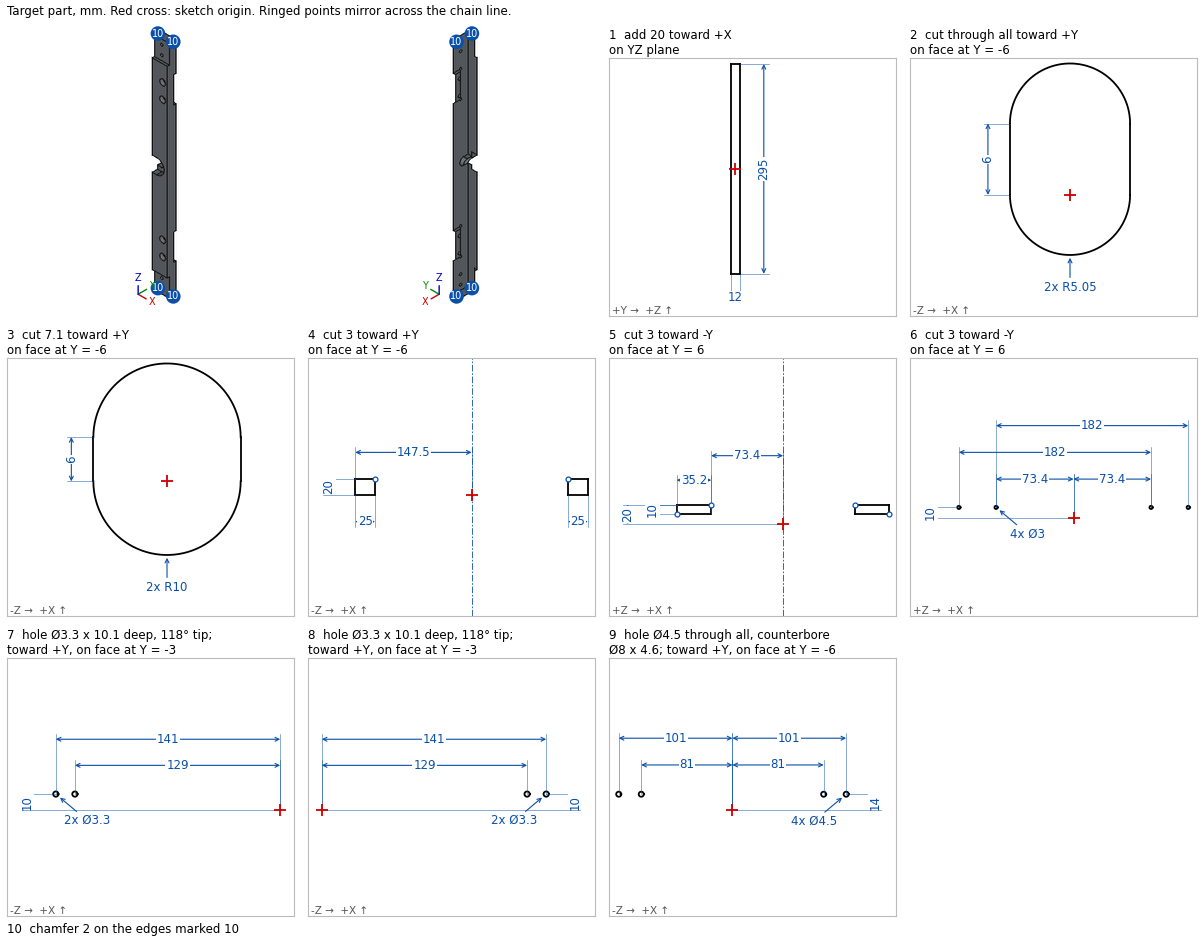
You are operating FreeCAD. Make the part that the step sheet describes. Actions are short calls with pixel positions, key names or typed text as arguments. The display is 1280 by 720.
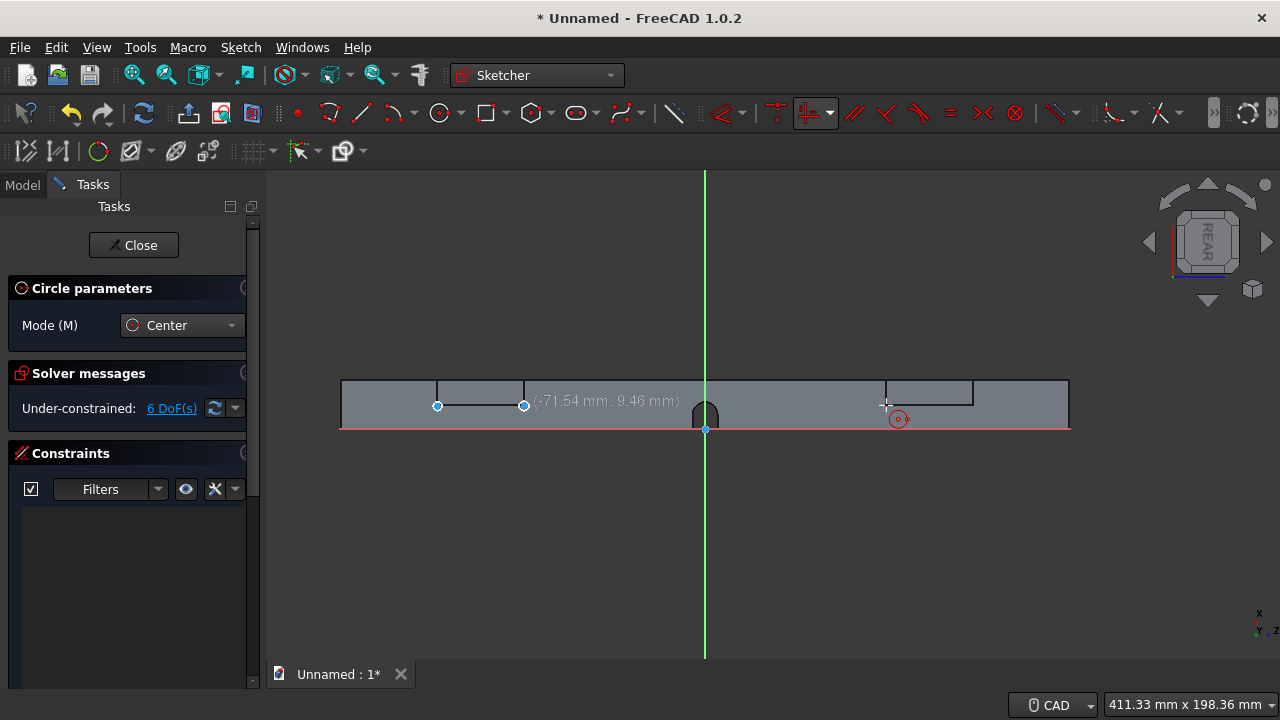
click(886, 405)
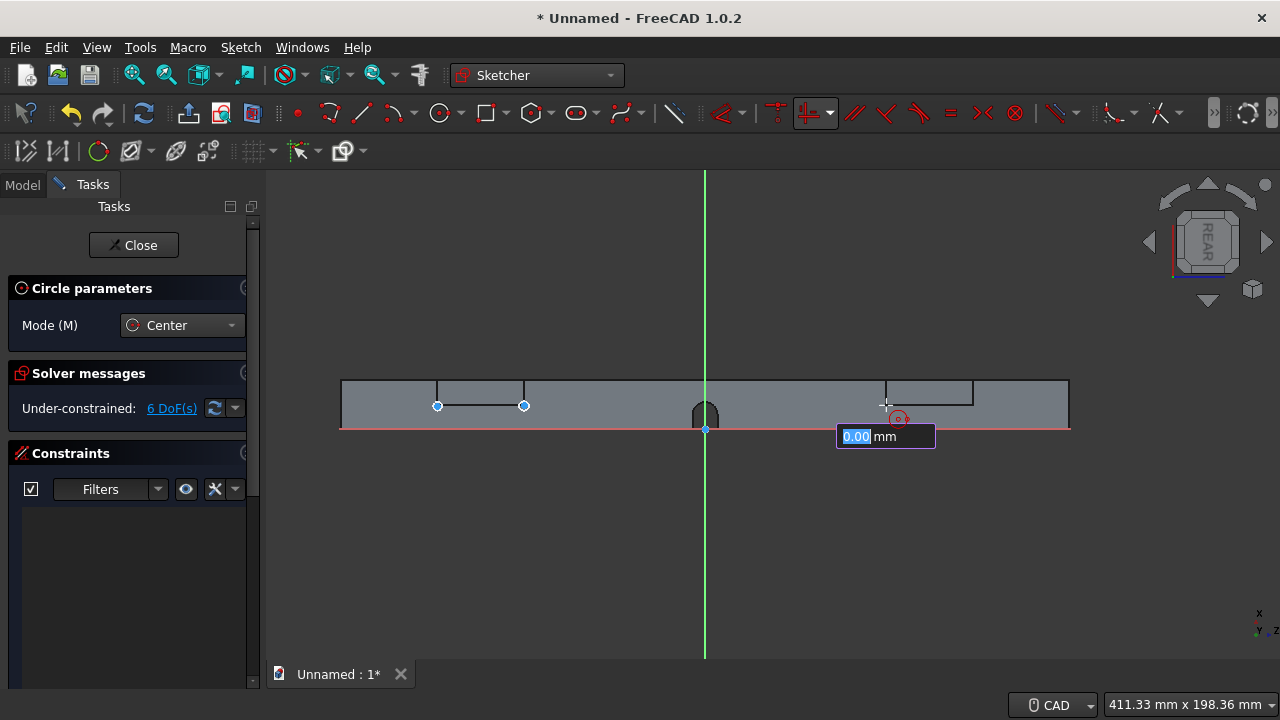
scroll(889, 402, up, 8)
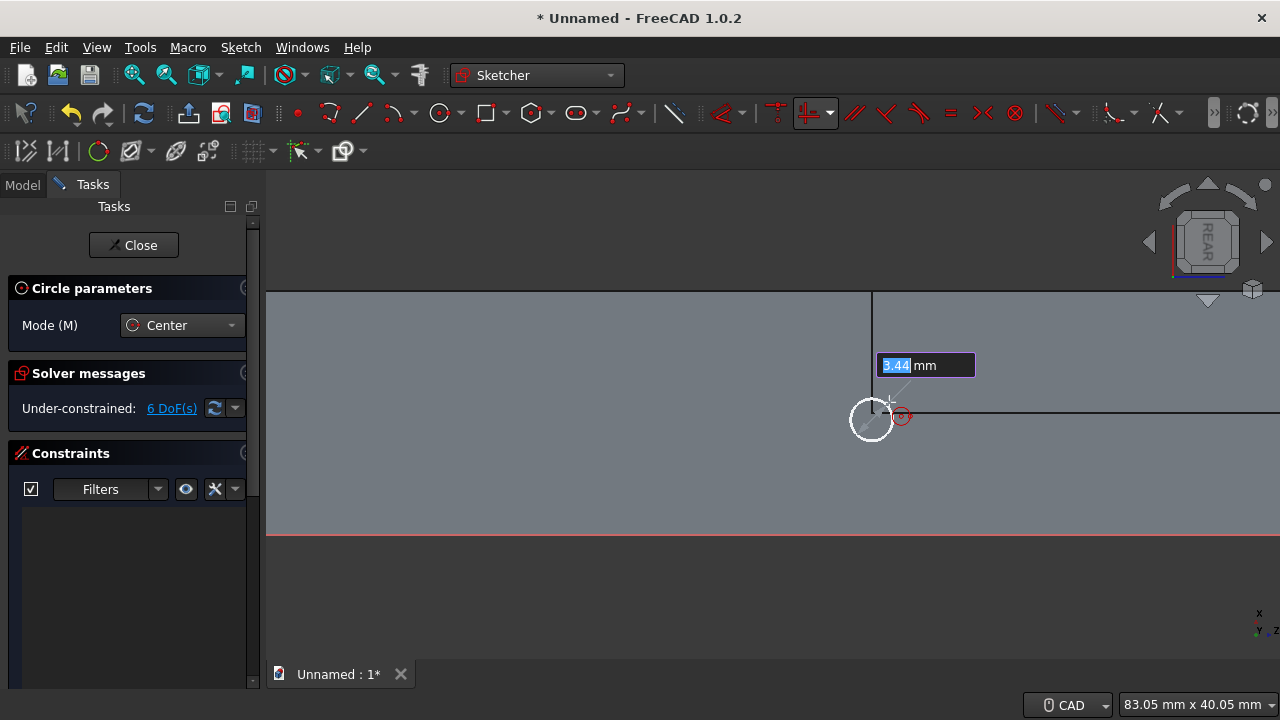
click(885, 400)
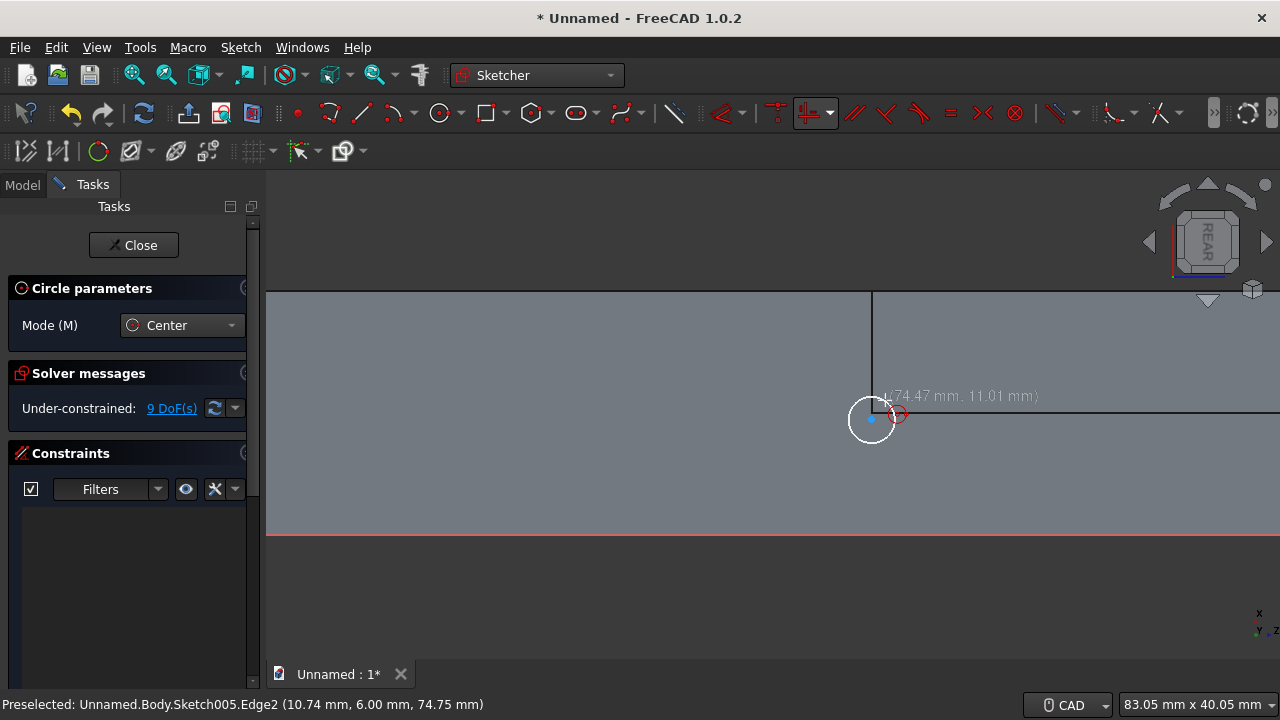
scroll(889, 402, down, 8)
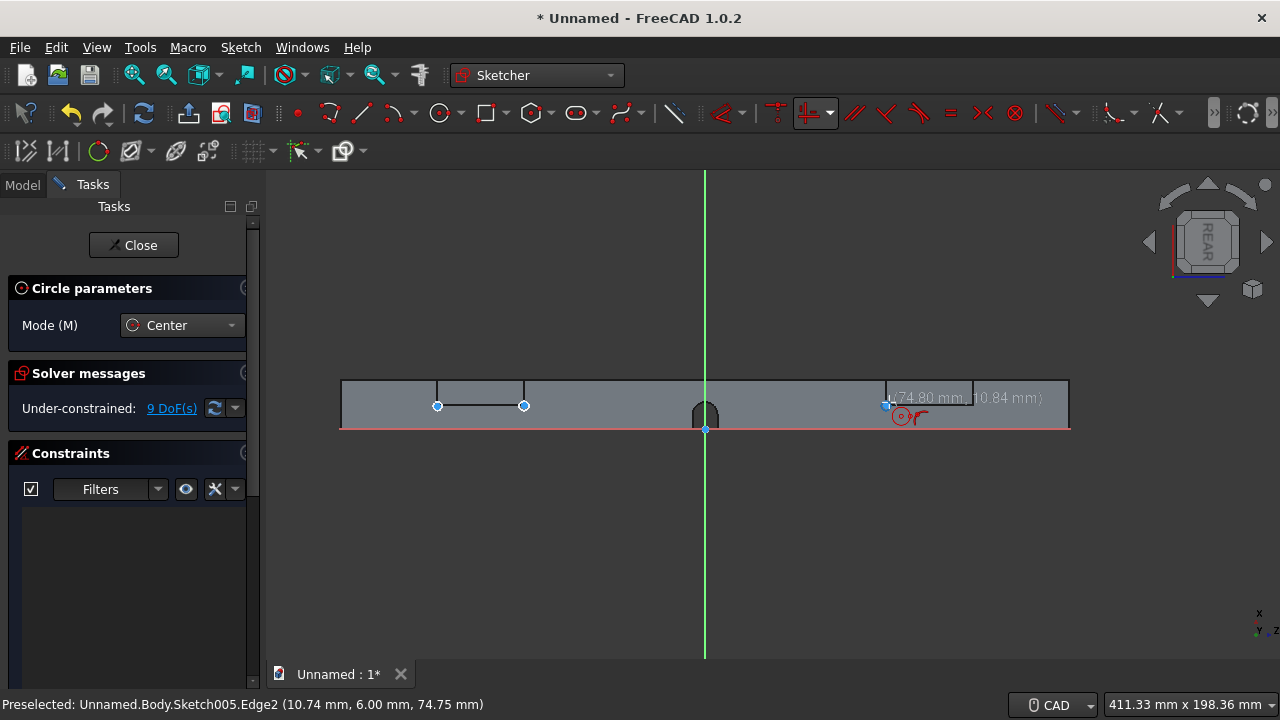
scroll(973, 405, up, 10)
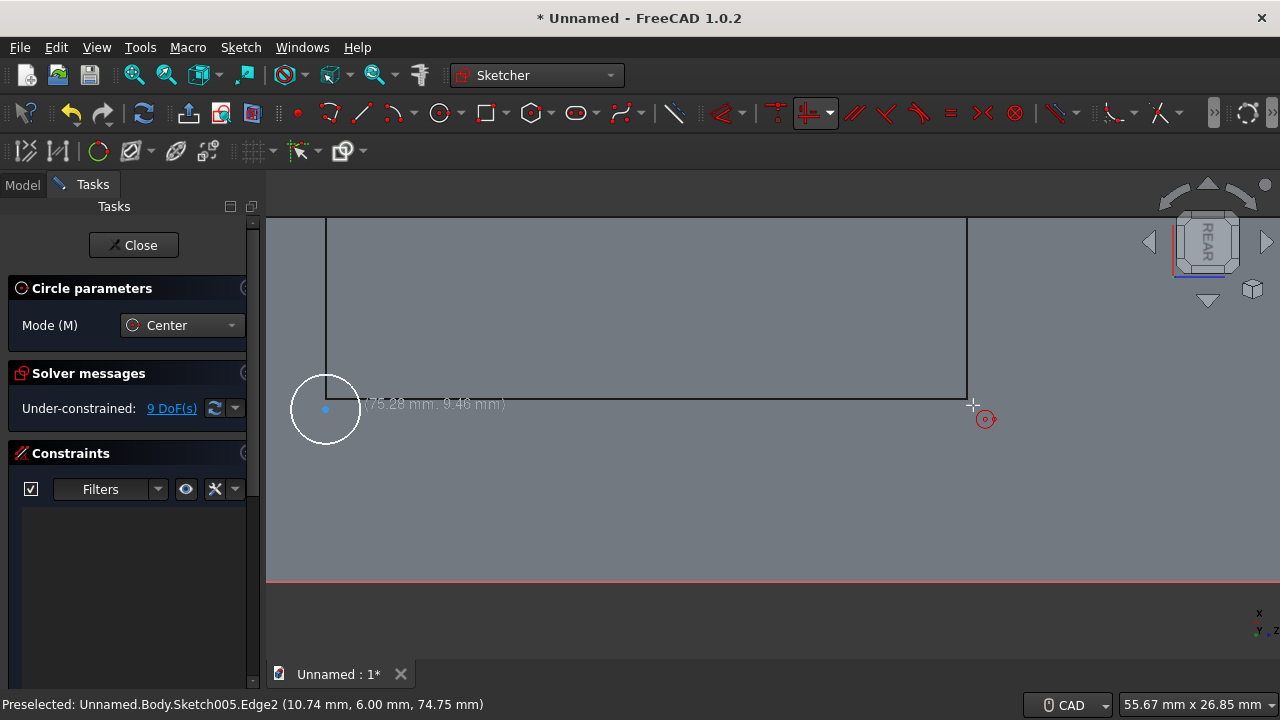
scroll(973, 405, down, 10)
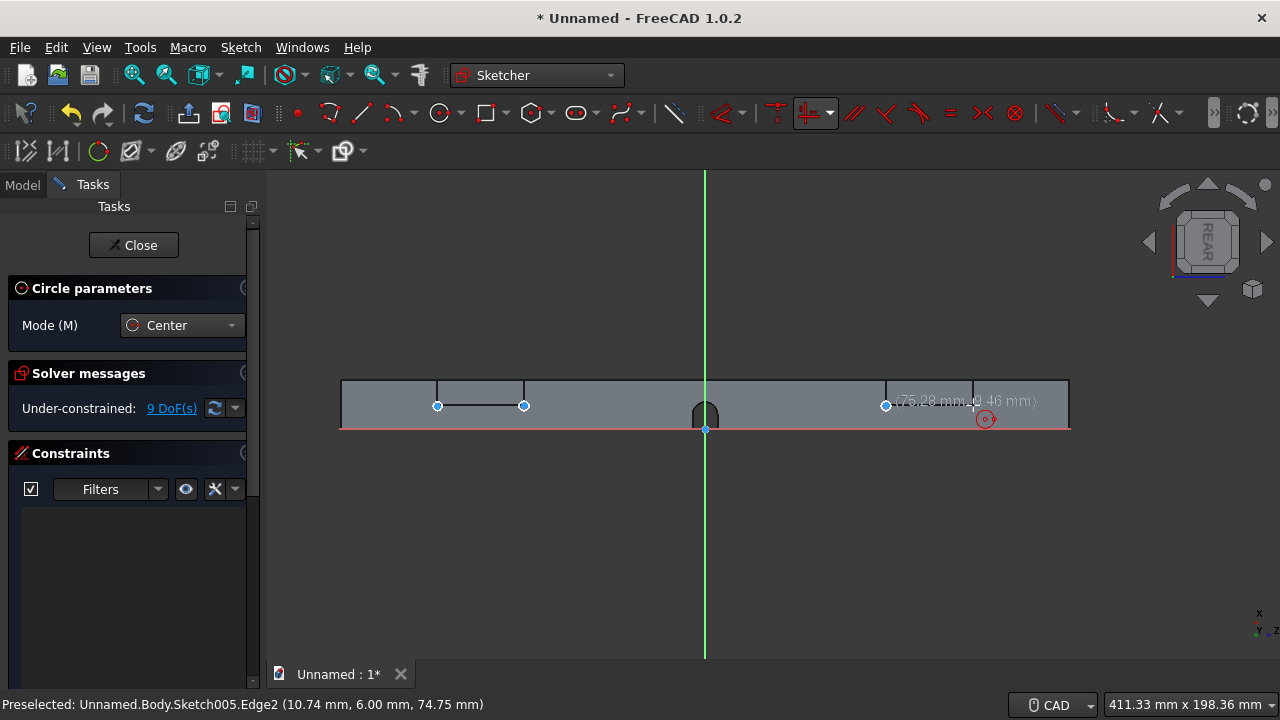
click(973, 405)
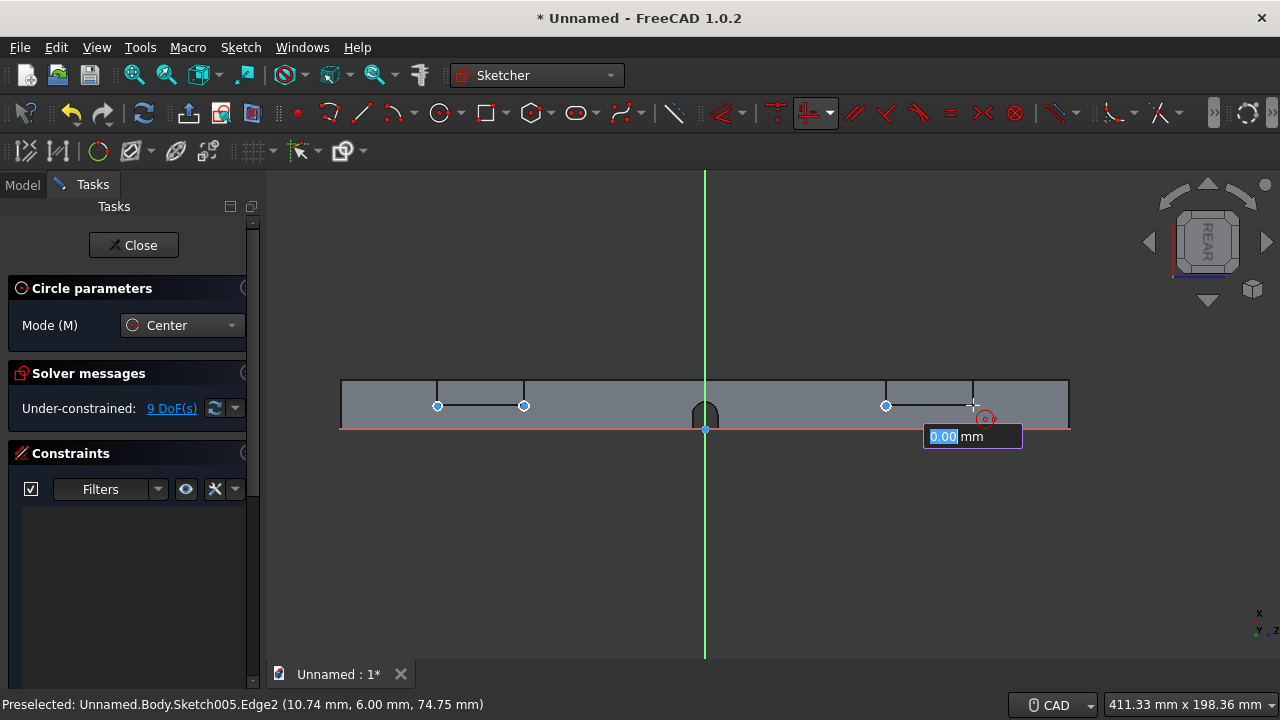
scroll(975, 402, up, 8)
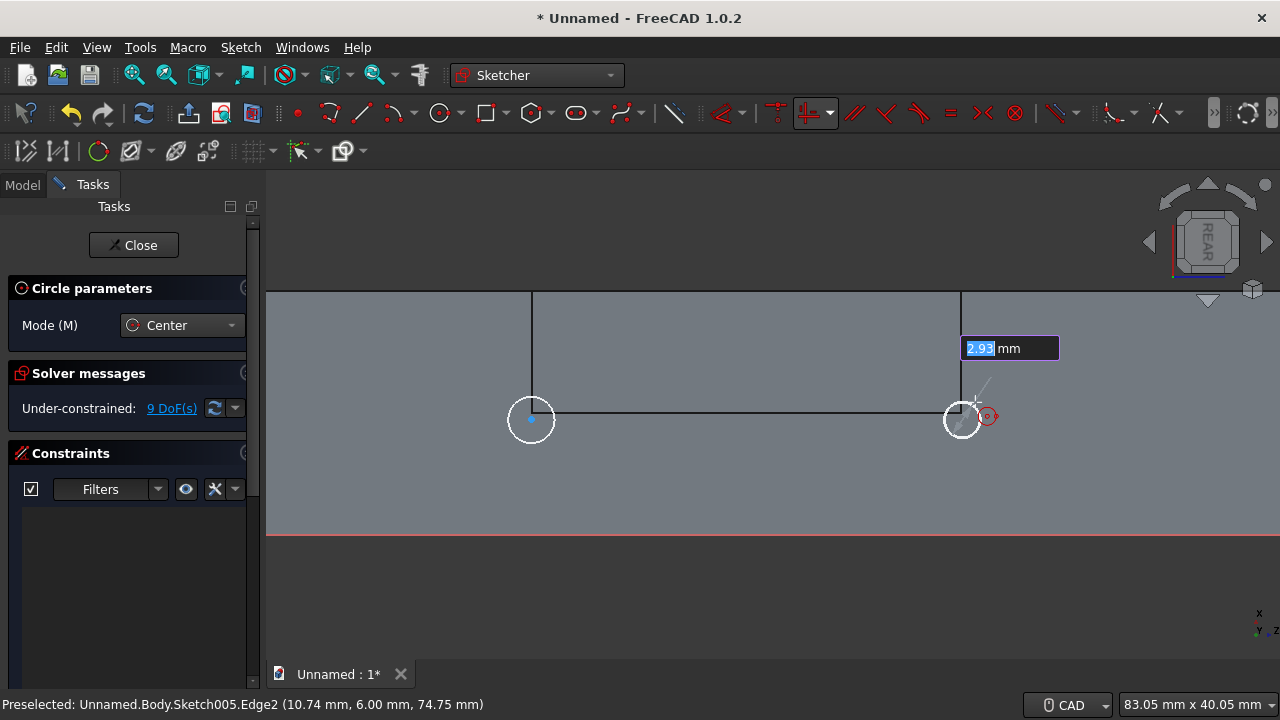
click(974, 400)
key(Escape)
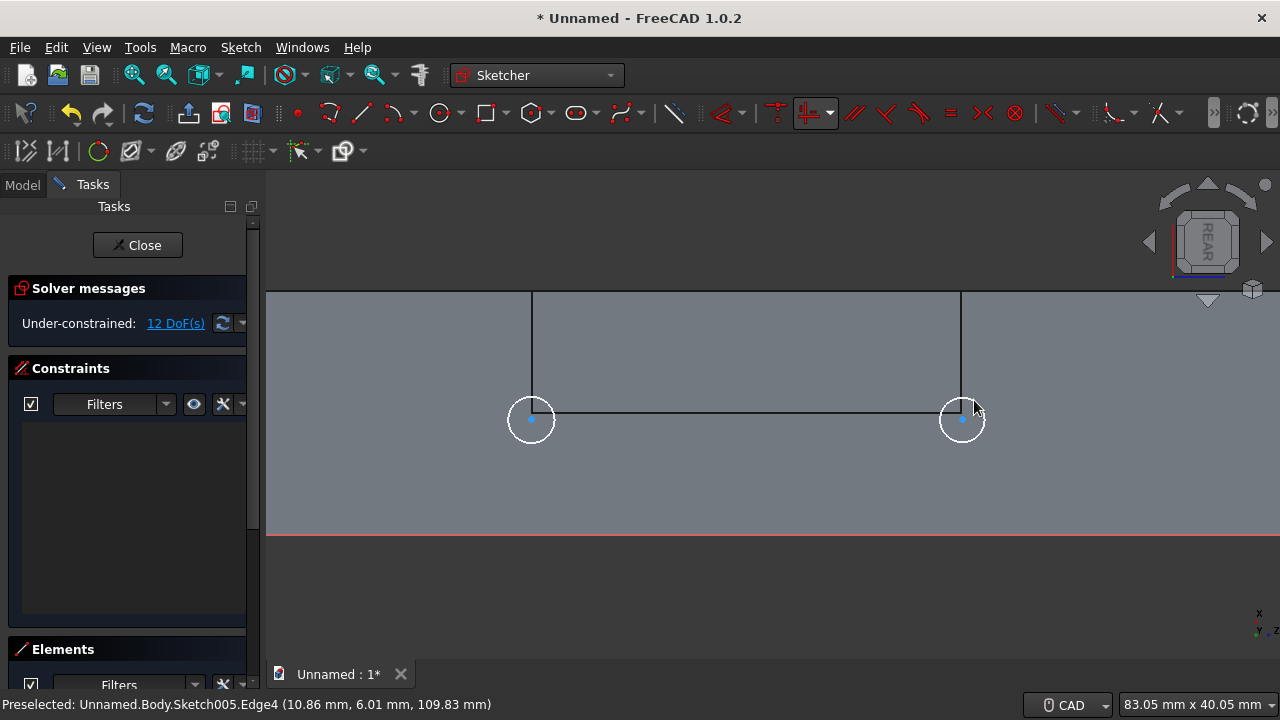
scroll(975, 402, down, 8)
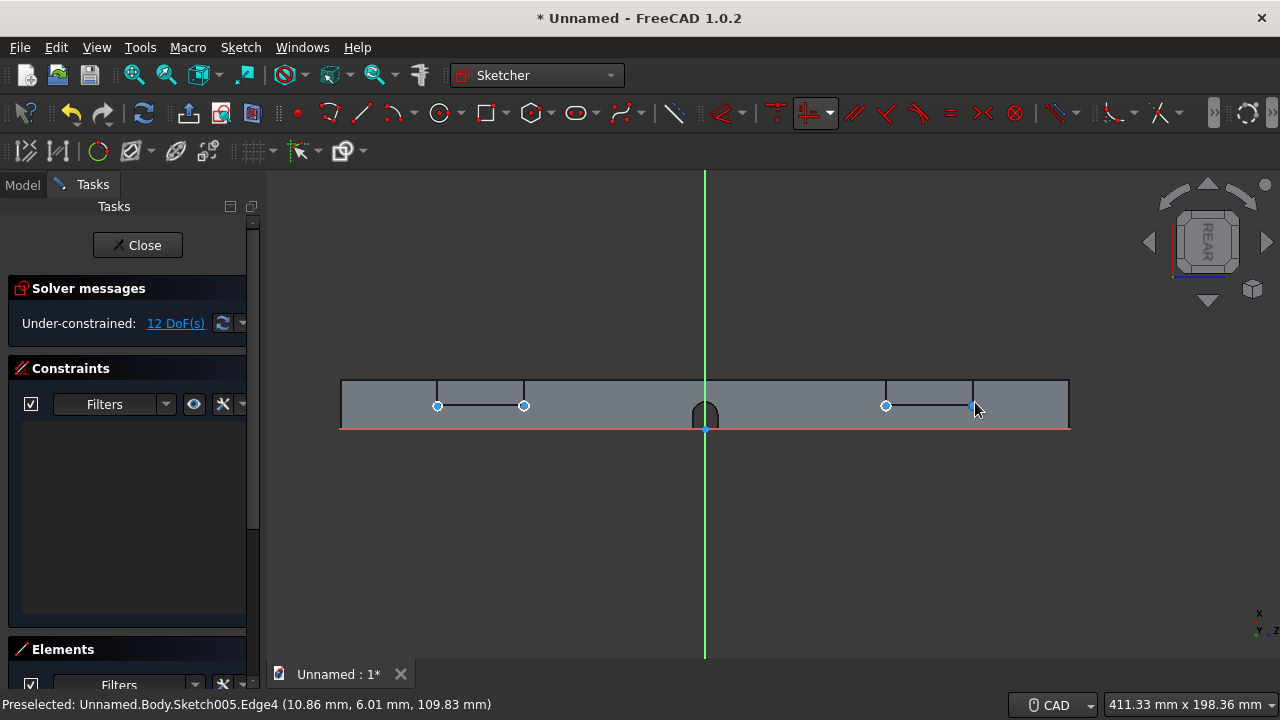
scroll(441, 403, up, 6)